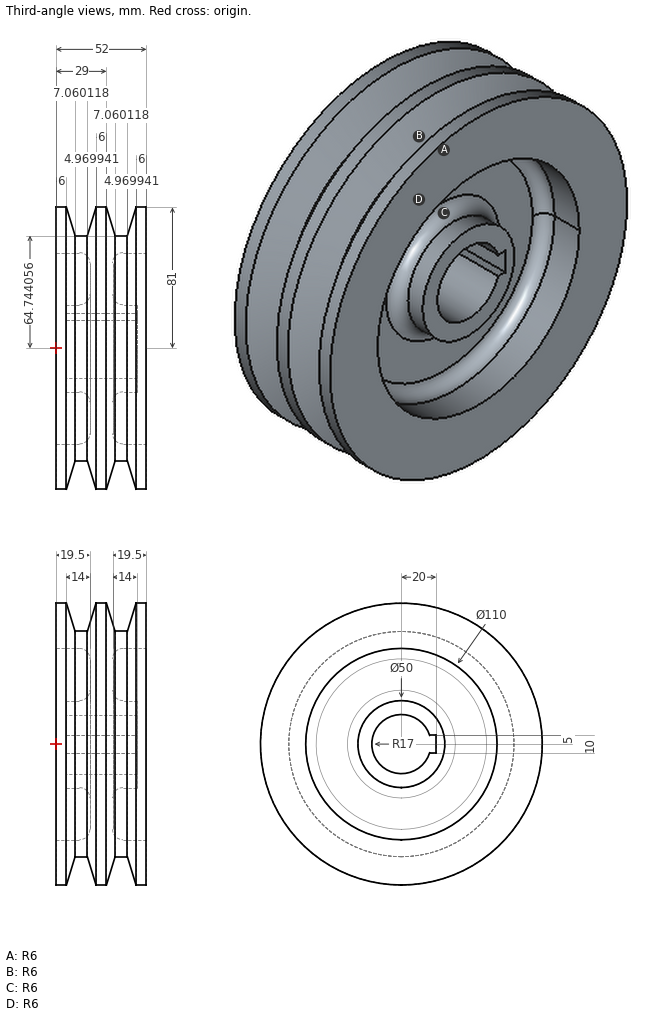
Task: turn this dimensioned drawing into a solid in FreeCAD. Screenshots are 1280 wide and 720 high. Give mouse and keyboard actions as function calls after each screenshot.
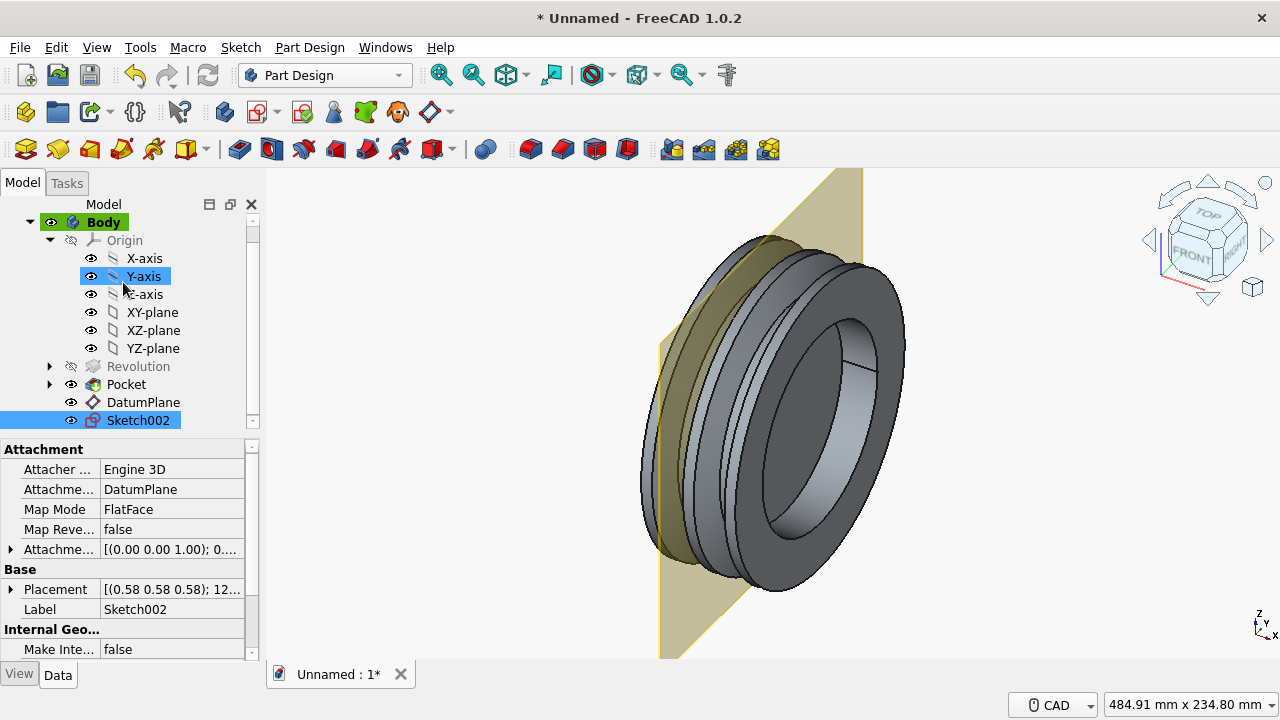
click(240, 150)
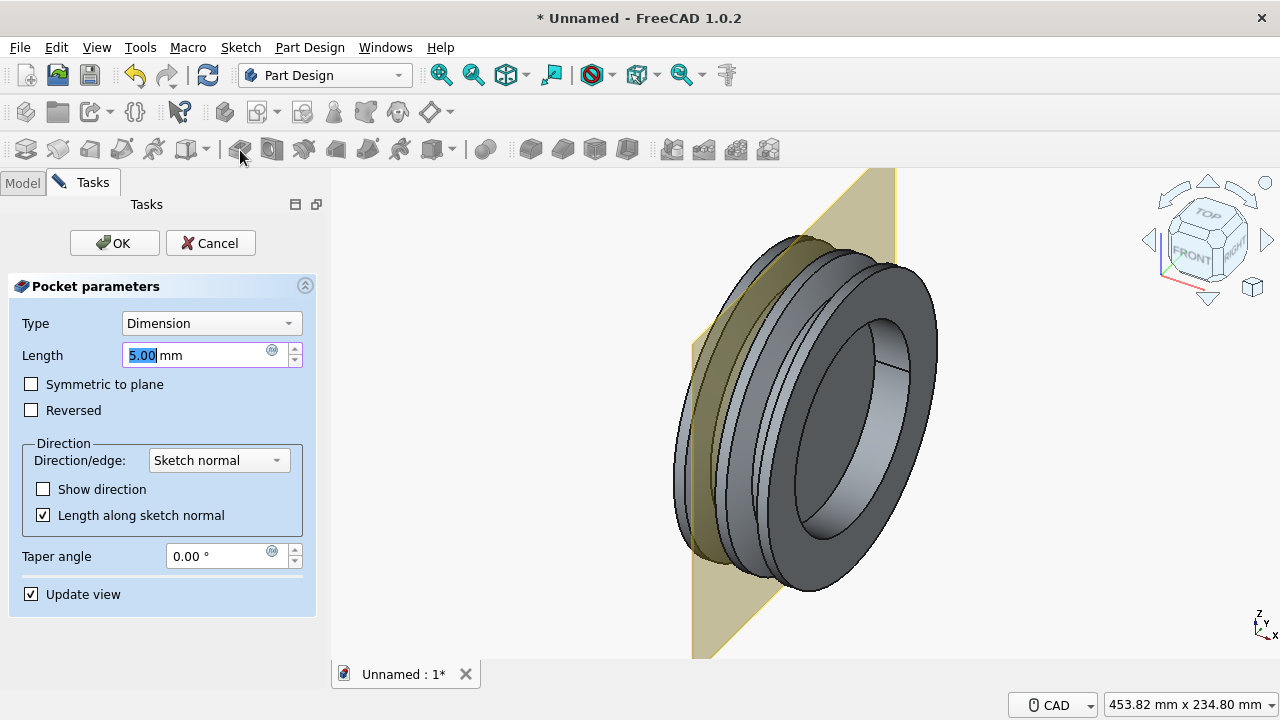
text(19.5)
key(Tab)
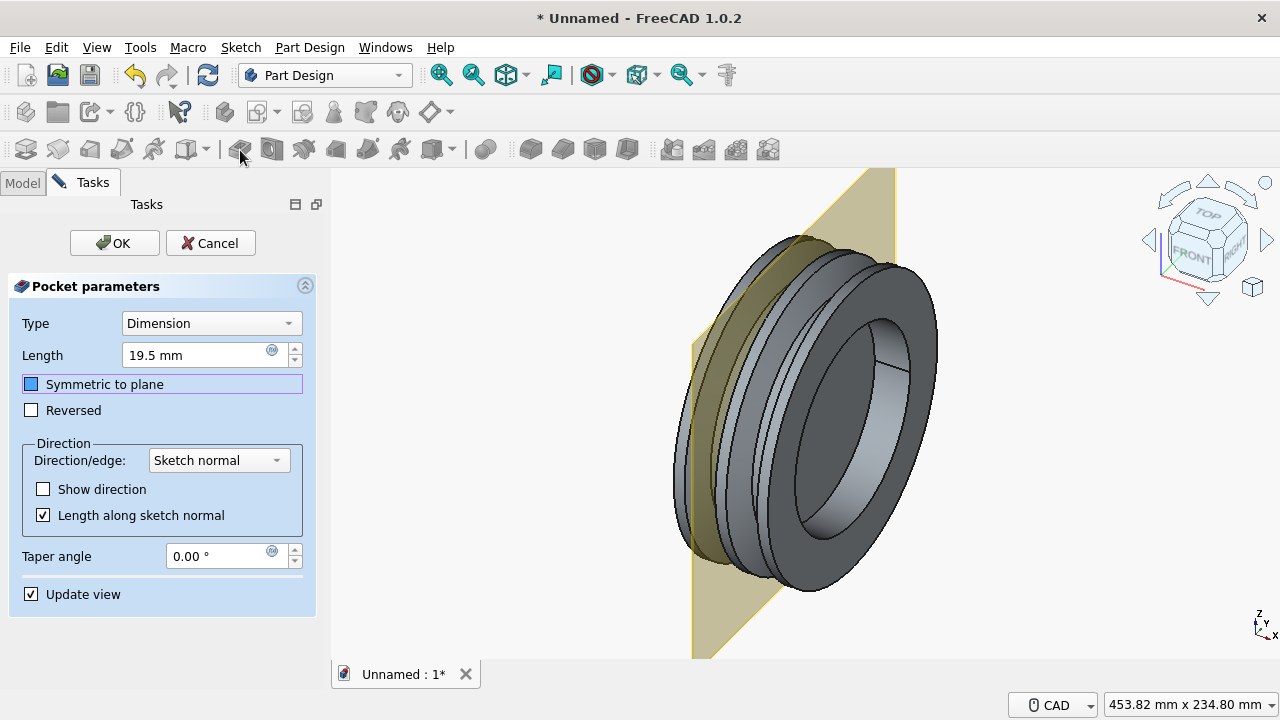
click(115, 243)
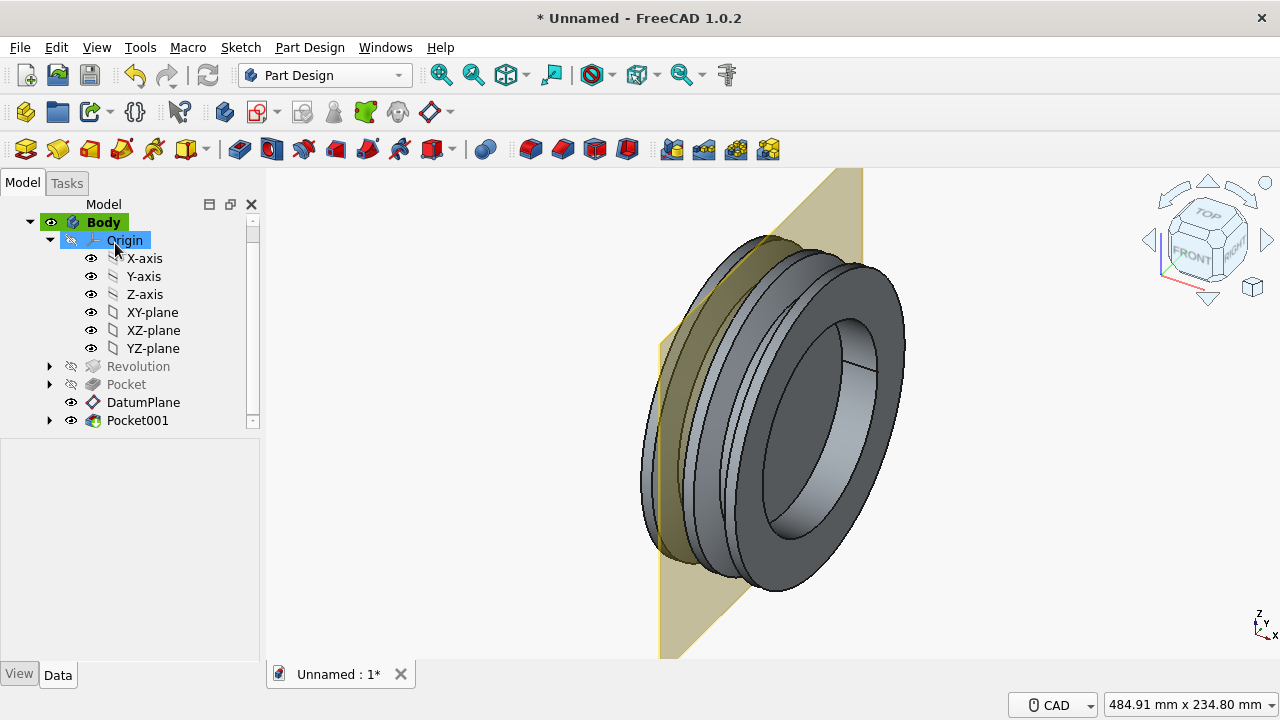
click(116, 402)
key(space)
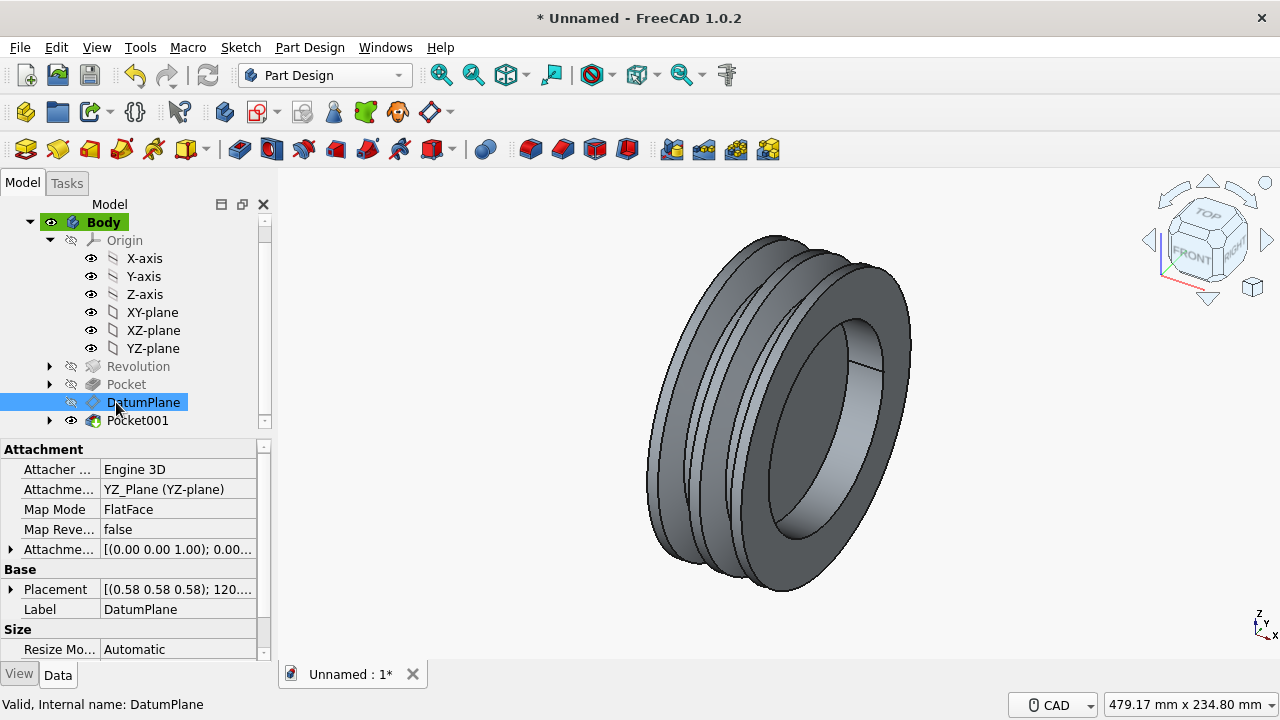
click(791, 416)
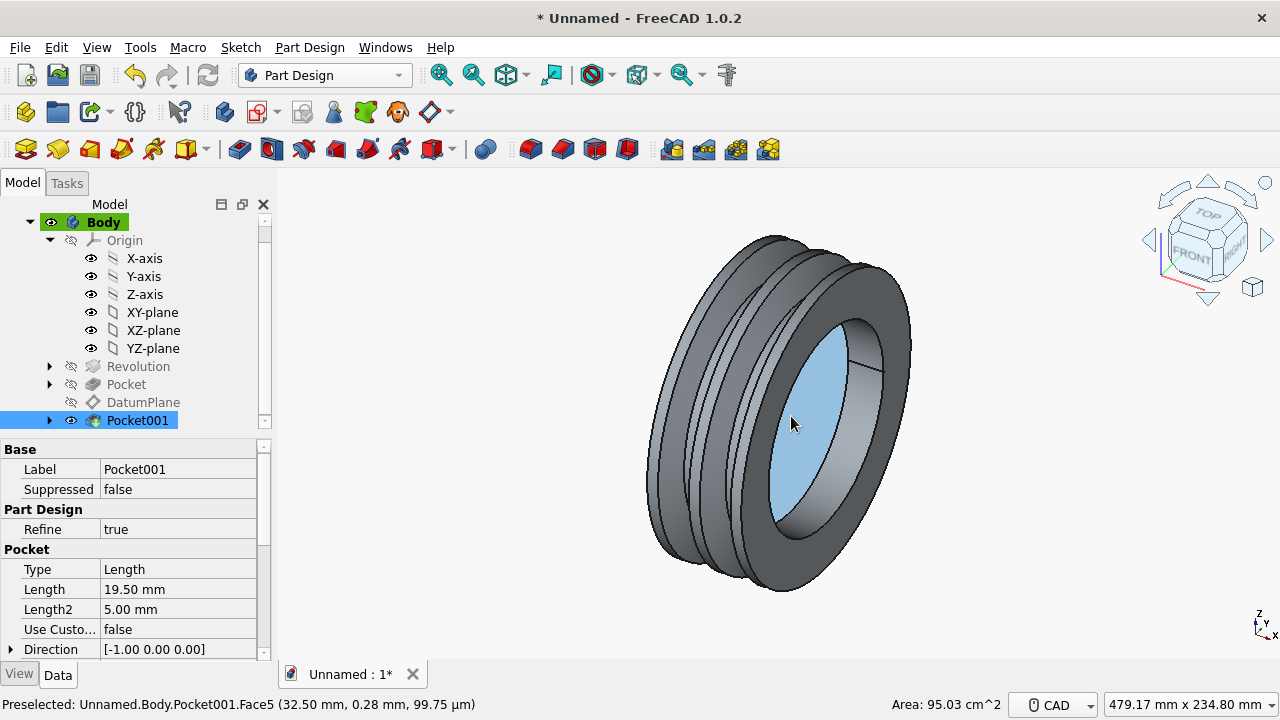
click(258, 112)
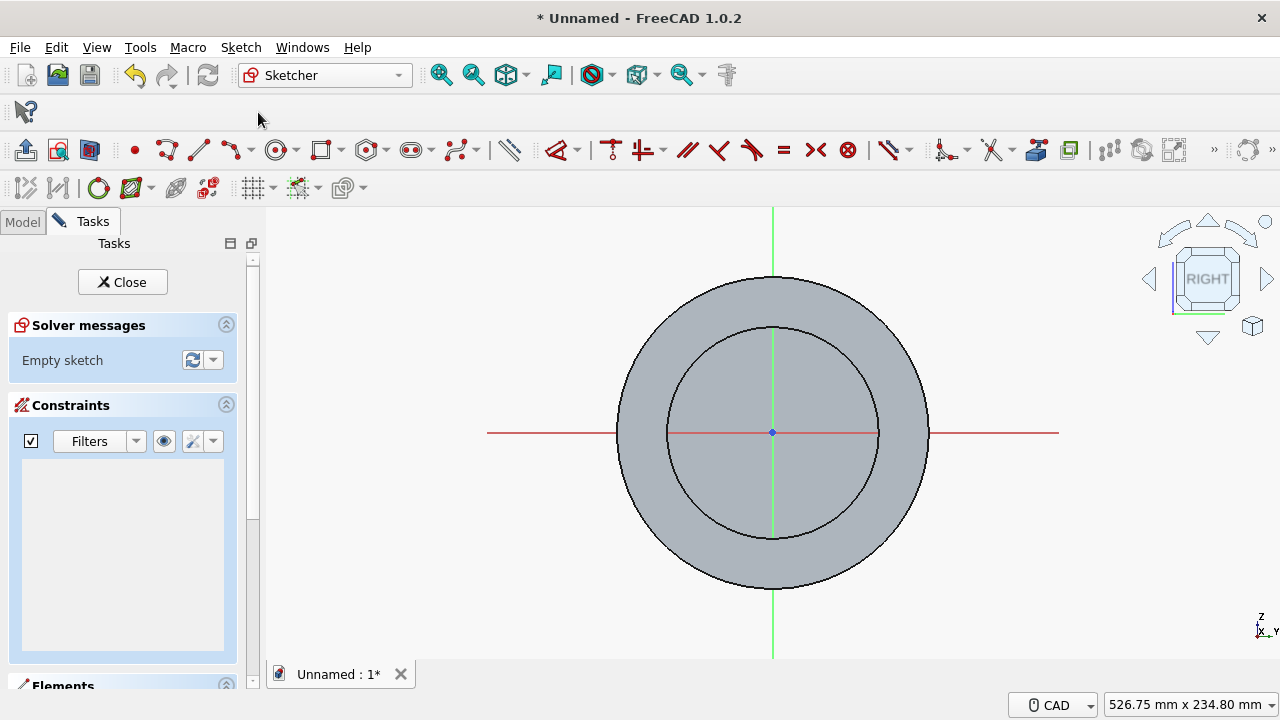
key(q)
key(s)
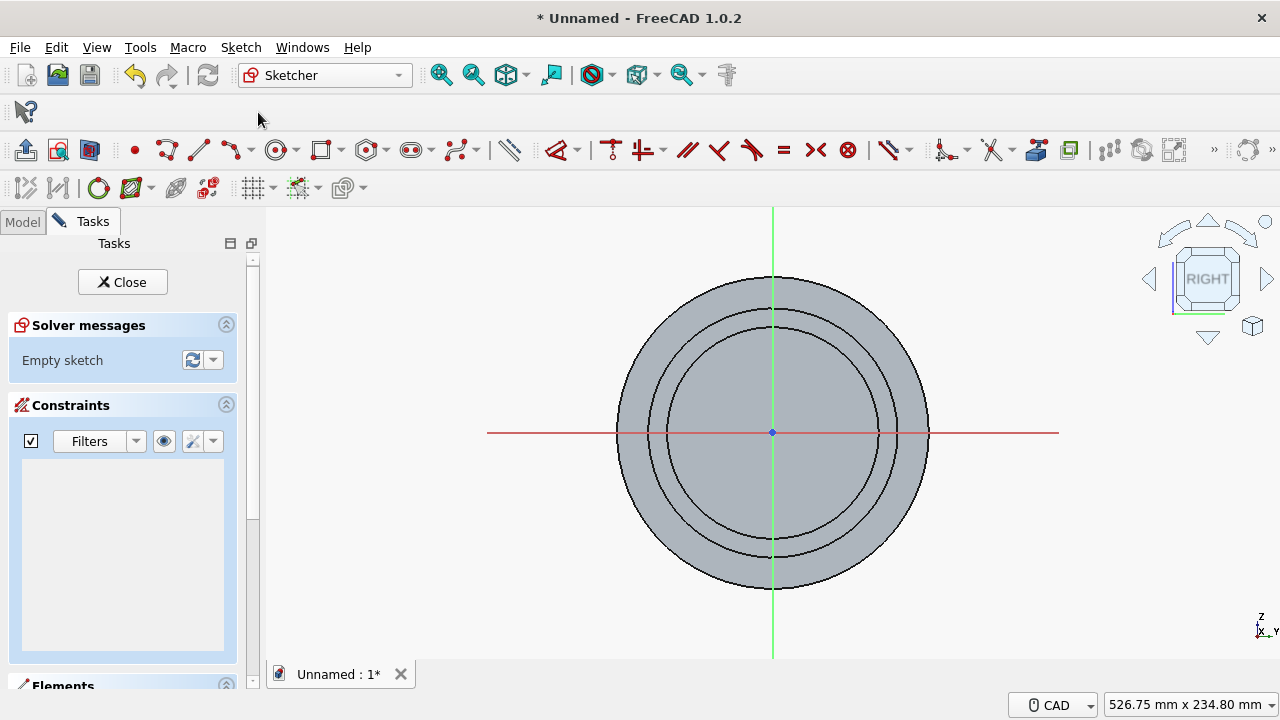
scroll(813, 433, up, 5)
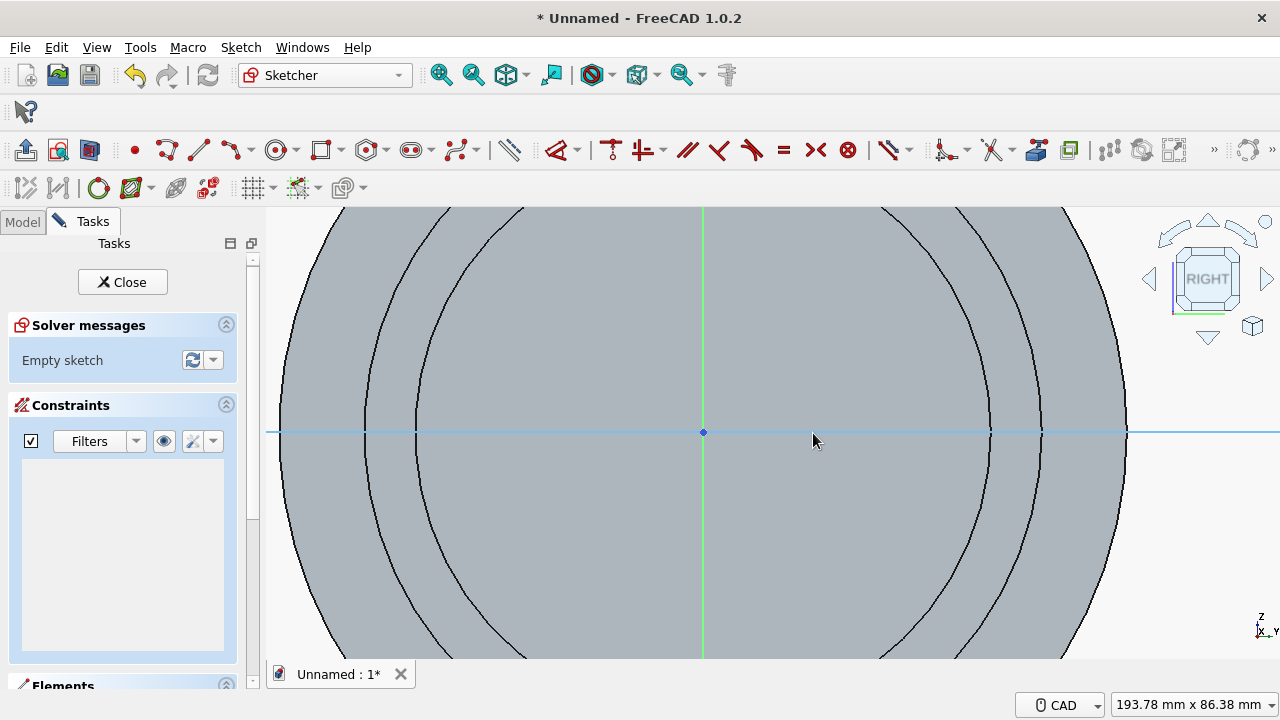
click(276, 150)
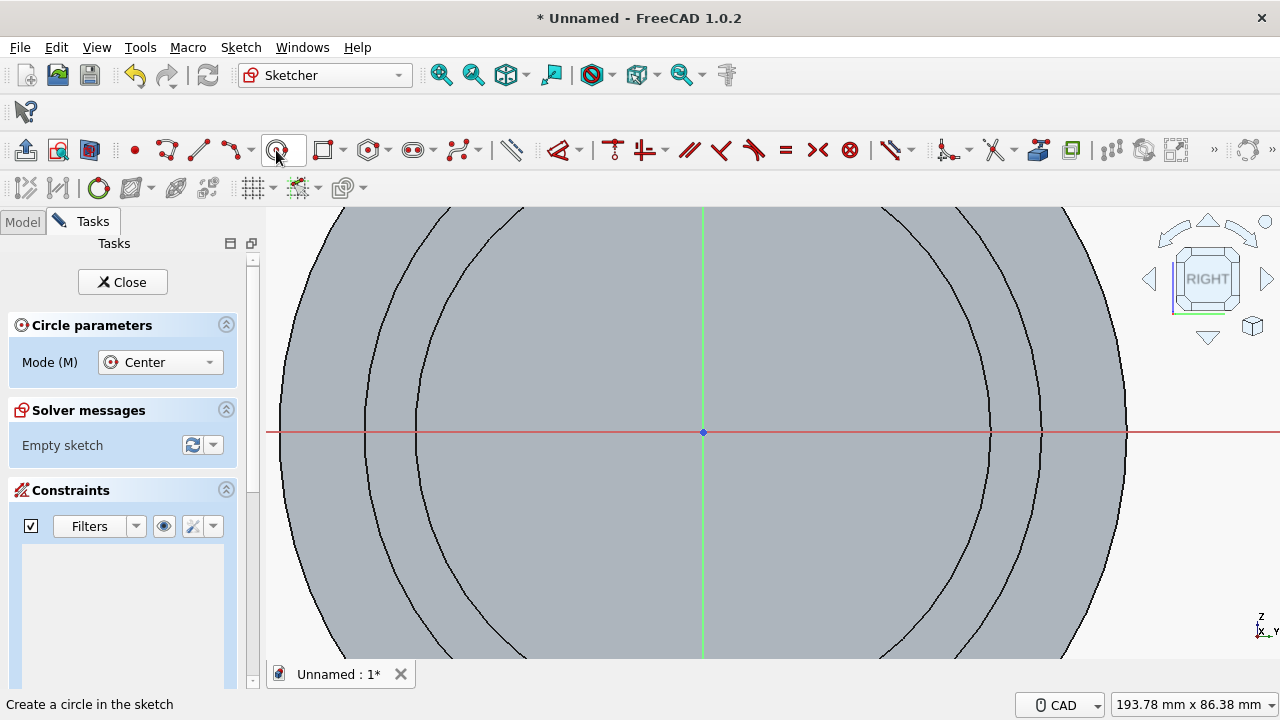
click(703, 432)
click(796, 340)
key(Escape)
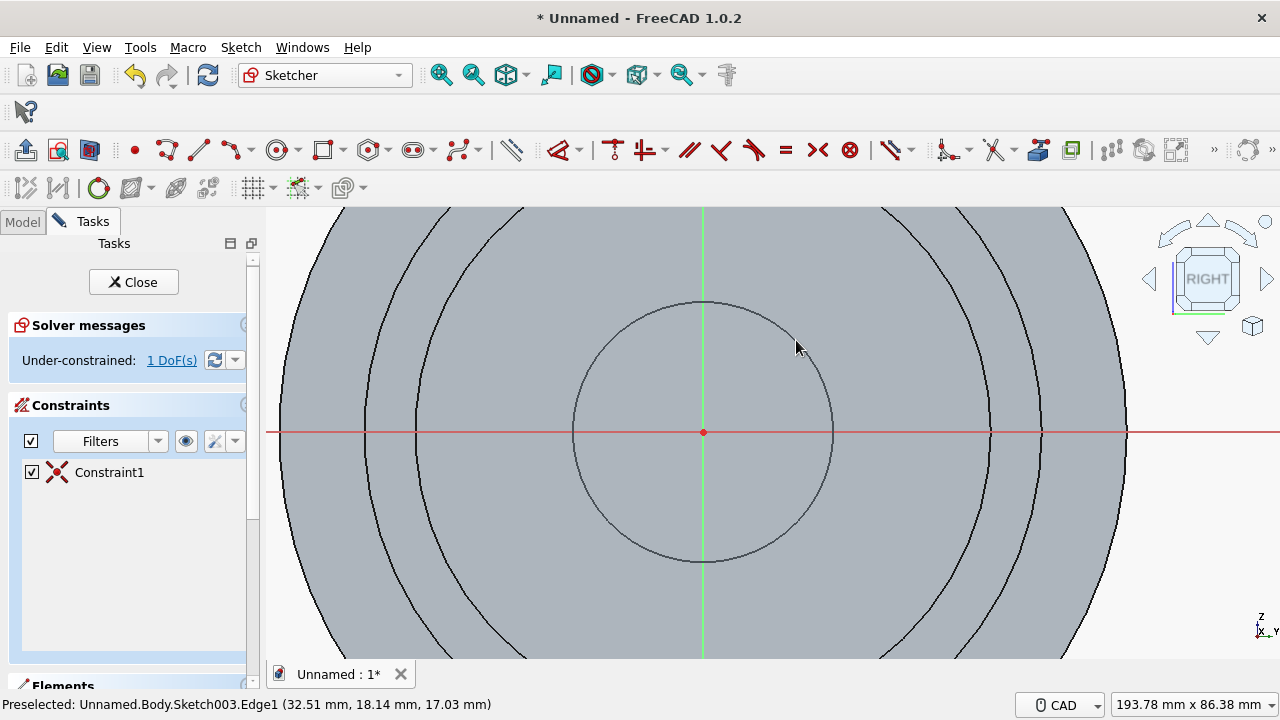
click(558, 150)